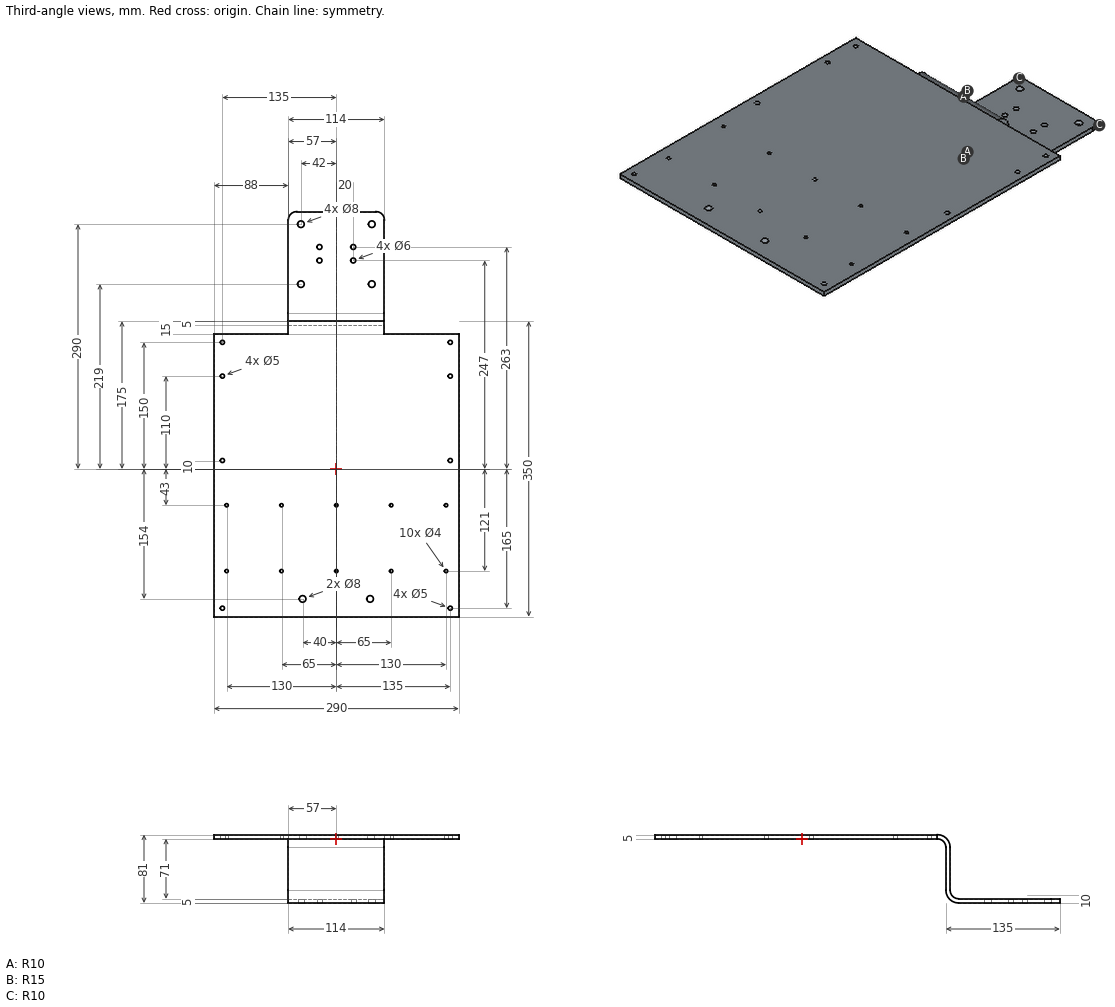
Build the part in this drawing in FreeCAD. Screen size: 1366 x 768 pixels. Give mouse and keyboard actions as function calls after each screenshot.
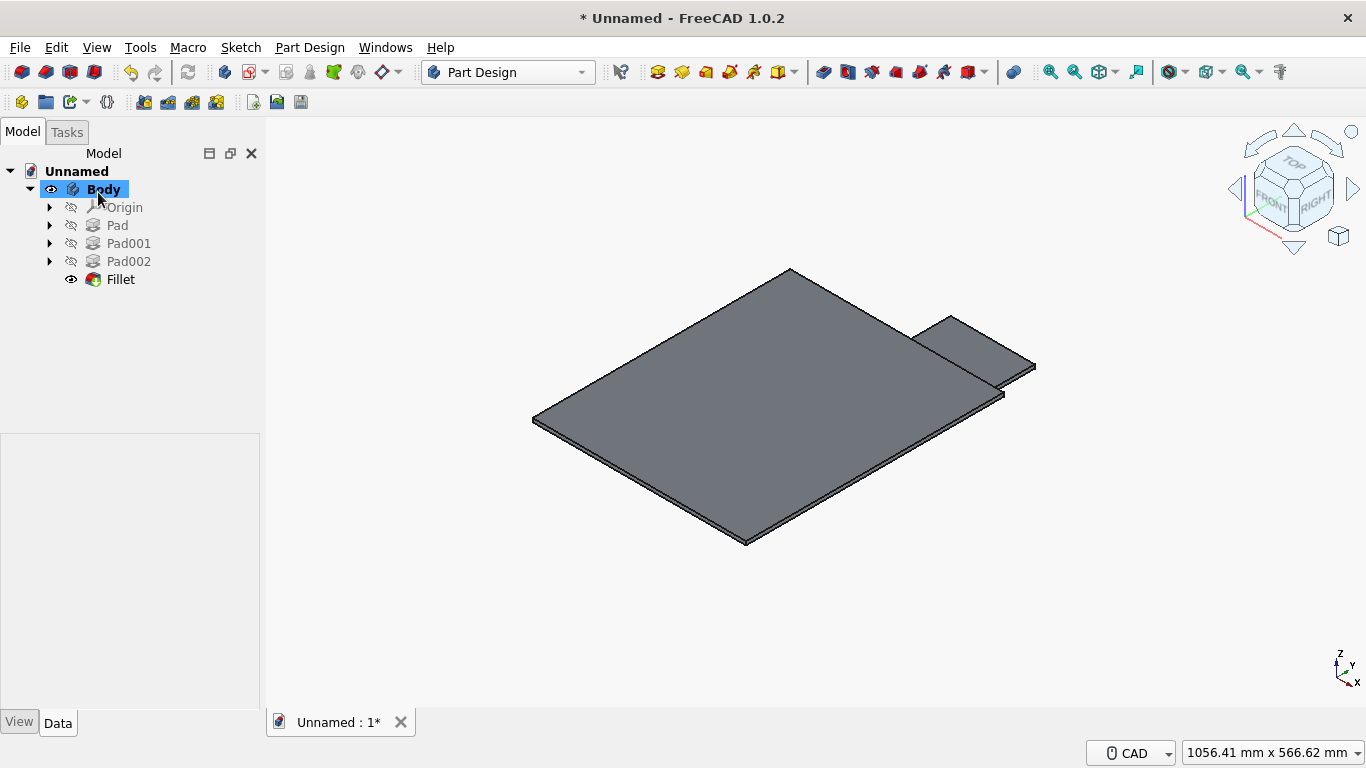
click(250, 72)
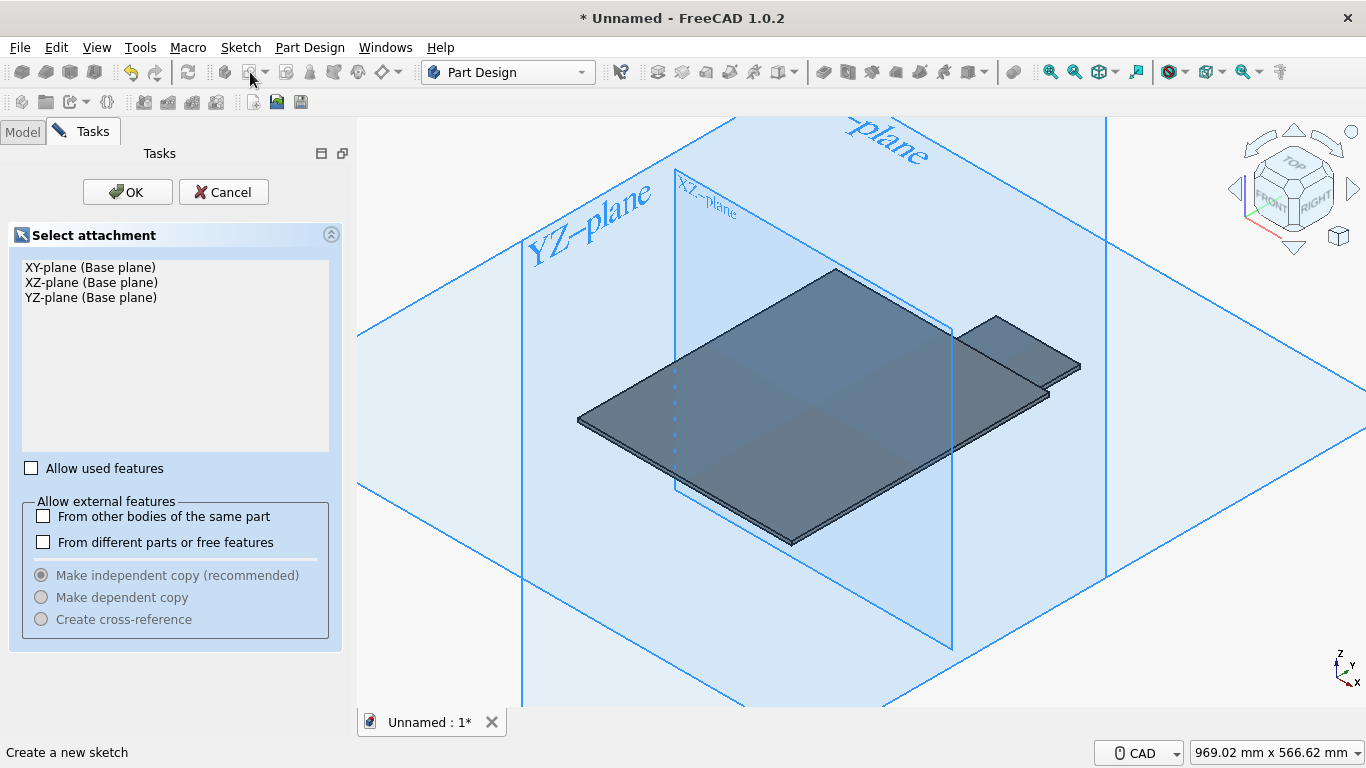
click(82, 268)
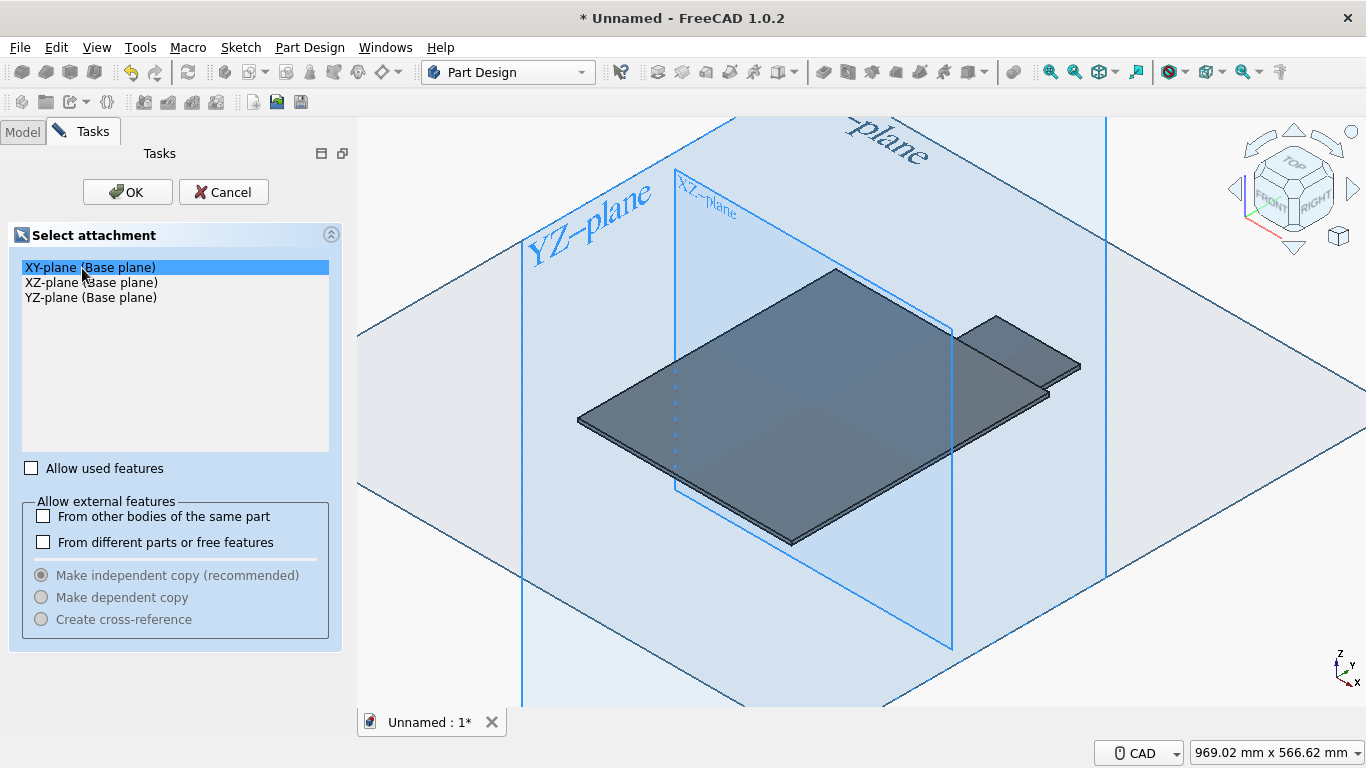
click(128, 192)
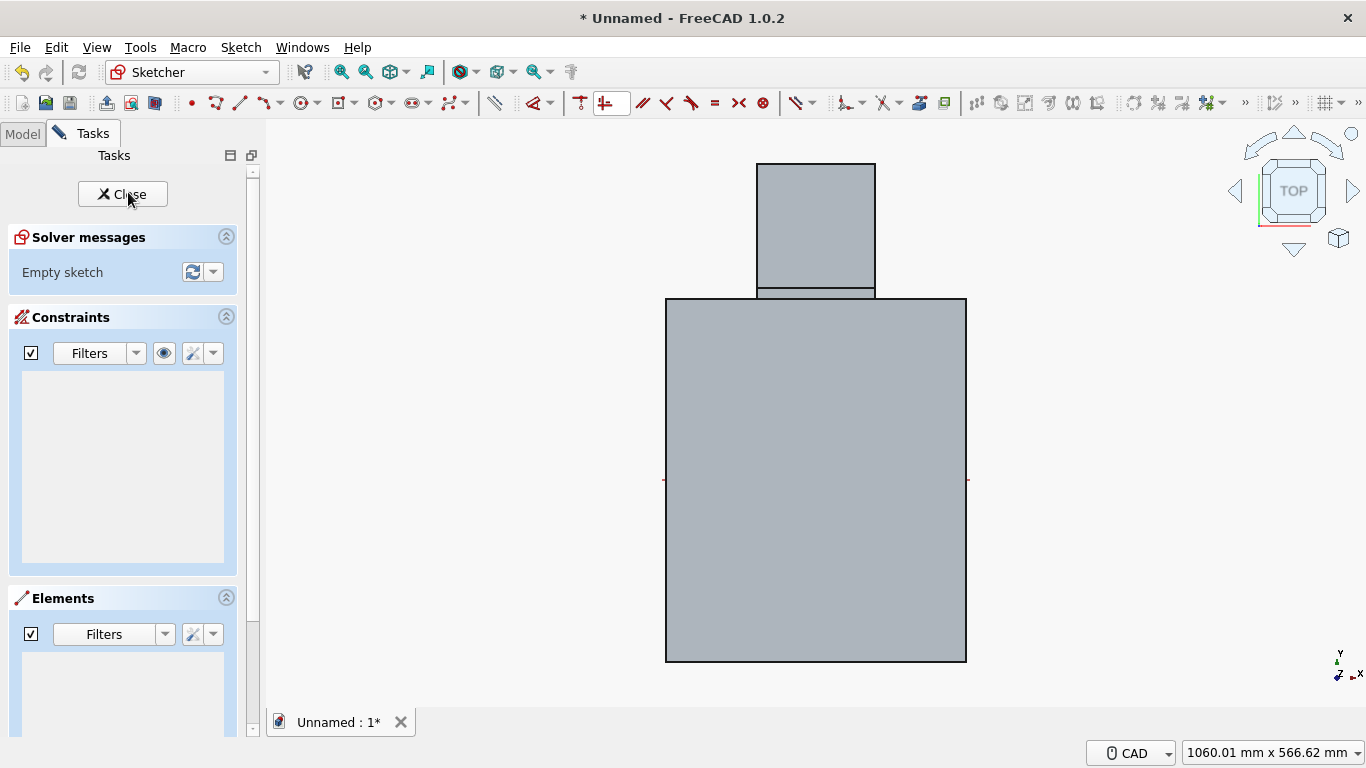
click(156, 104)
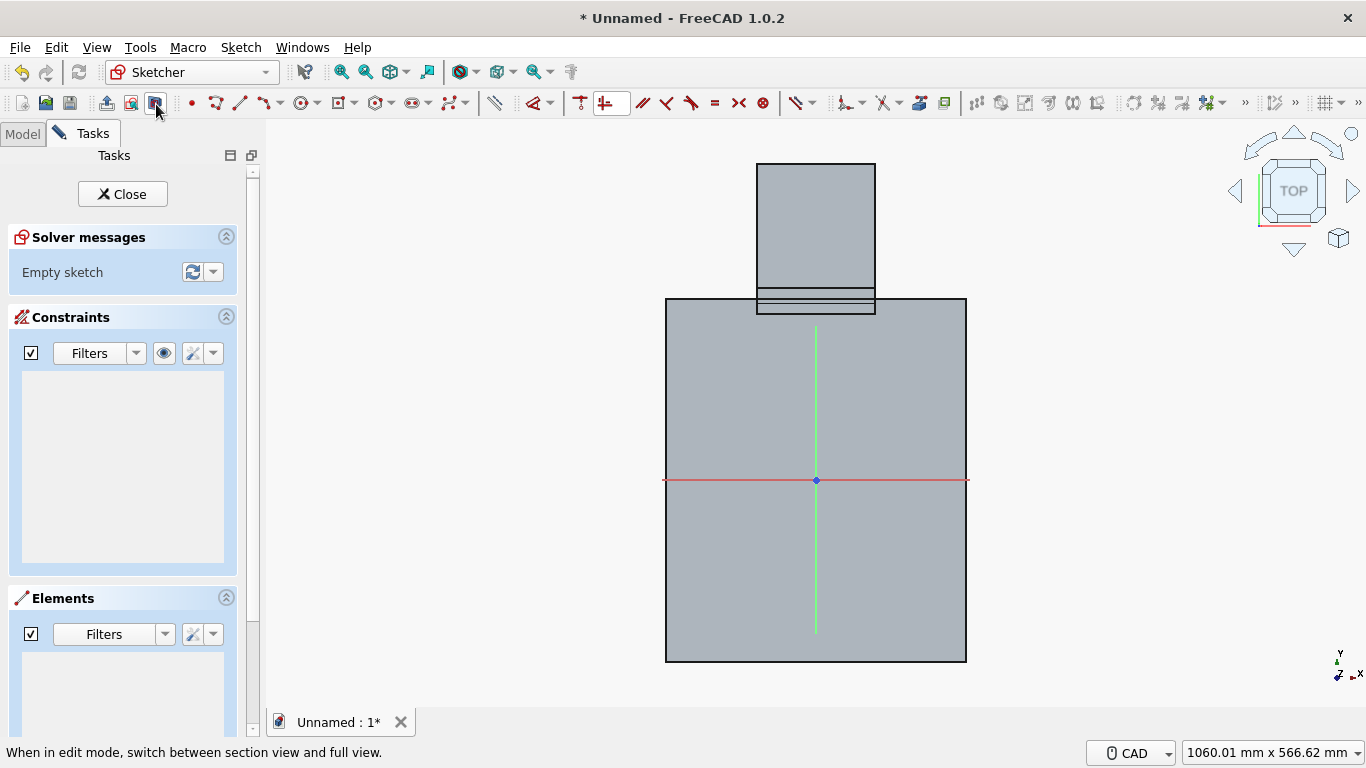
scroll(872, 371, up, 4)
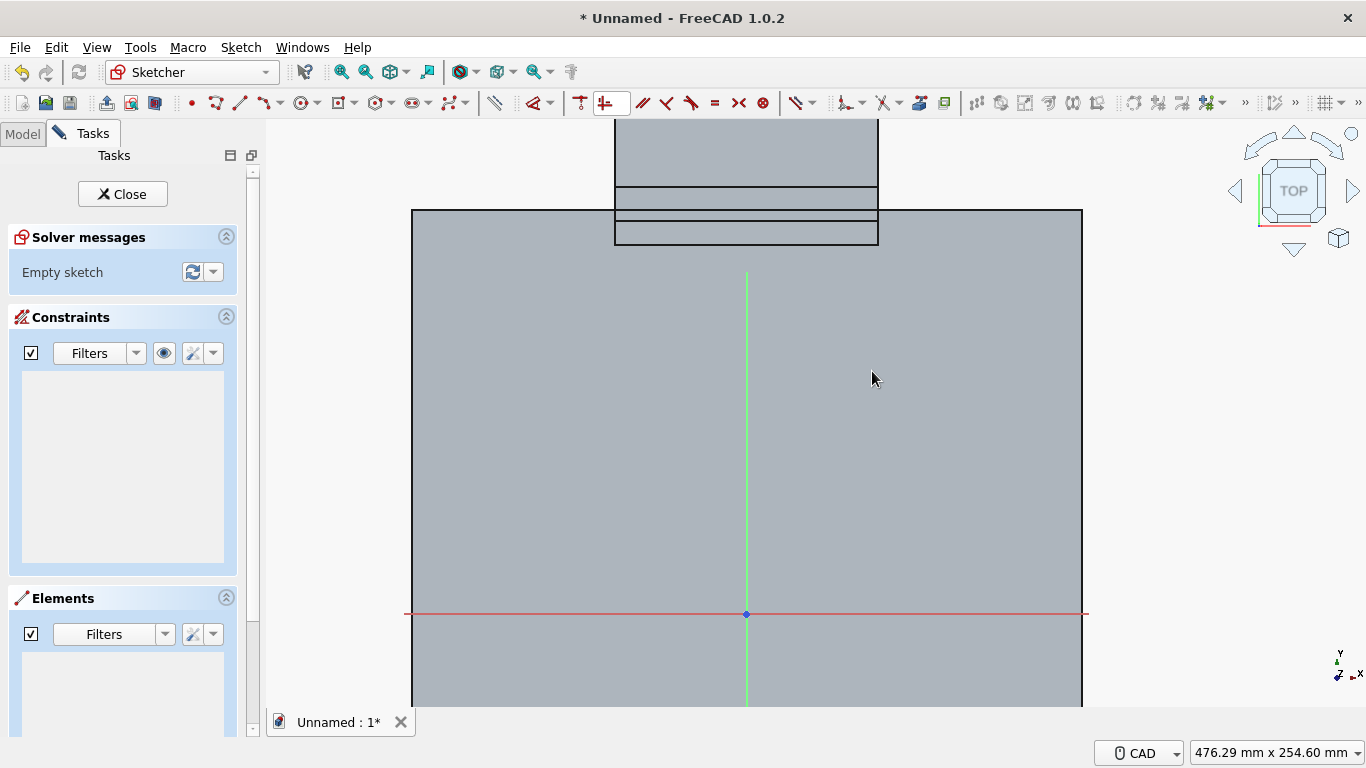
key(g)
key(r)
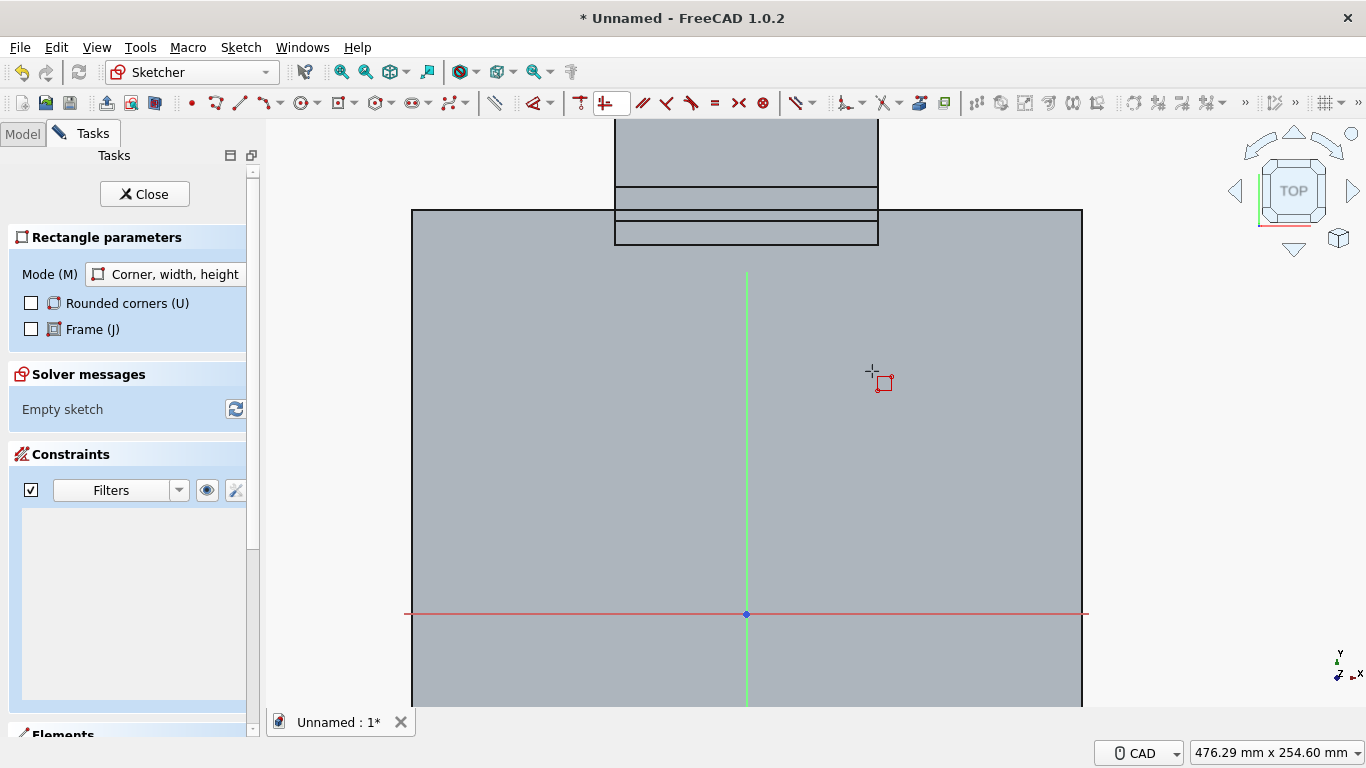
click(412, 210)
click(615, 245)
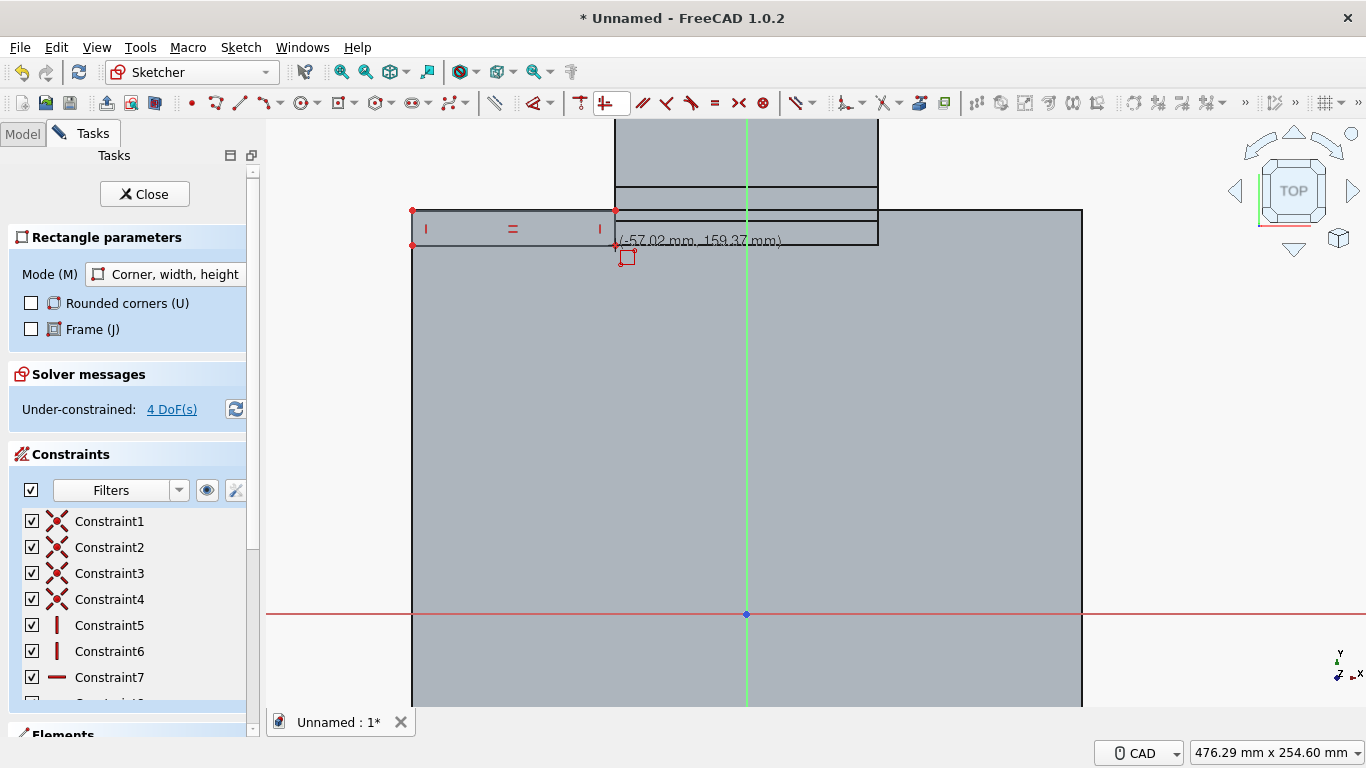
click(878, 210)
click(1082, 245)
key(Escape)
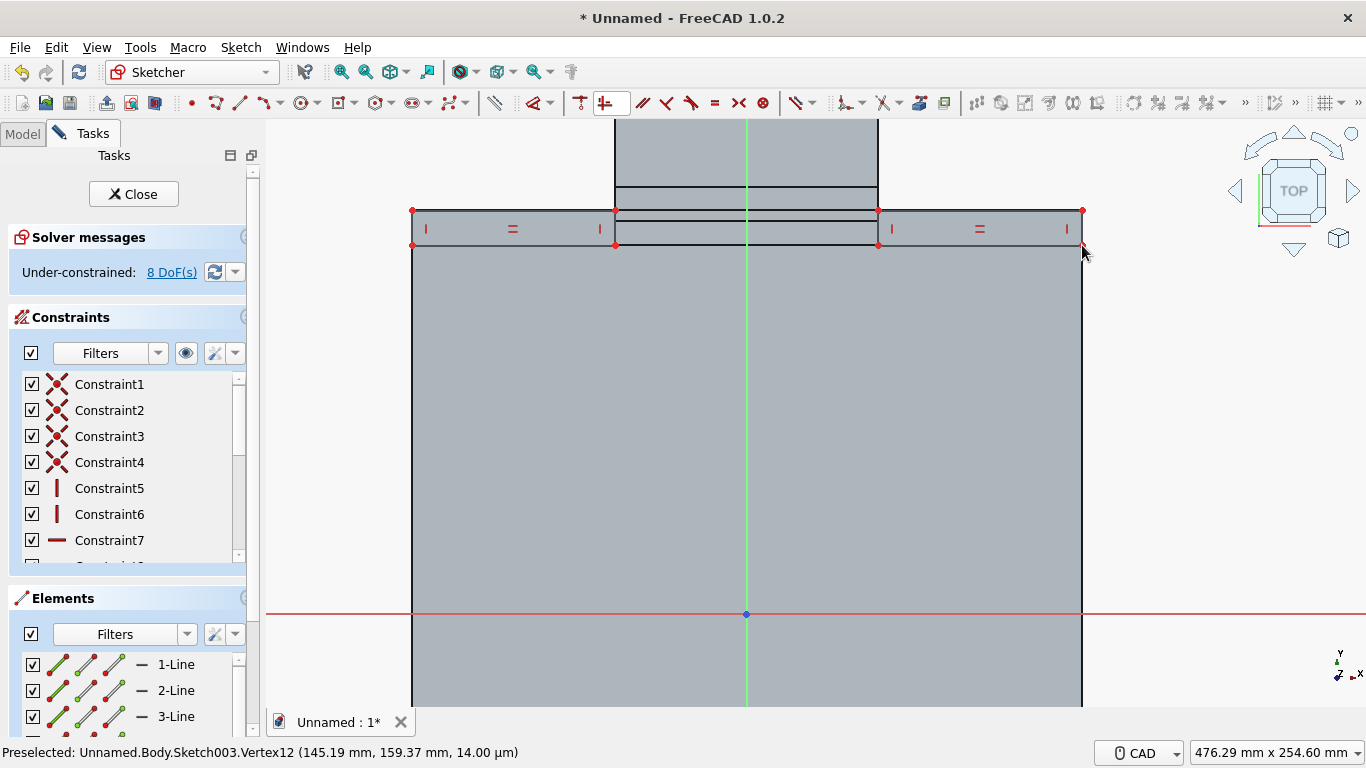
click(615, 211)